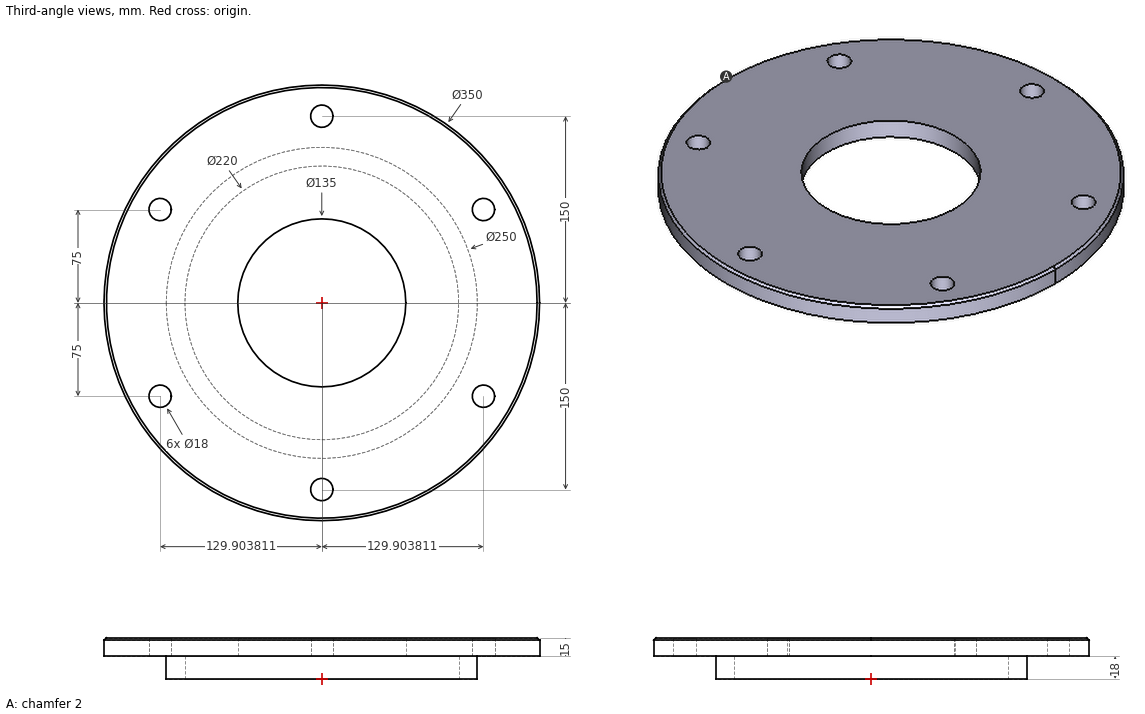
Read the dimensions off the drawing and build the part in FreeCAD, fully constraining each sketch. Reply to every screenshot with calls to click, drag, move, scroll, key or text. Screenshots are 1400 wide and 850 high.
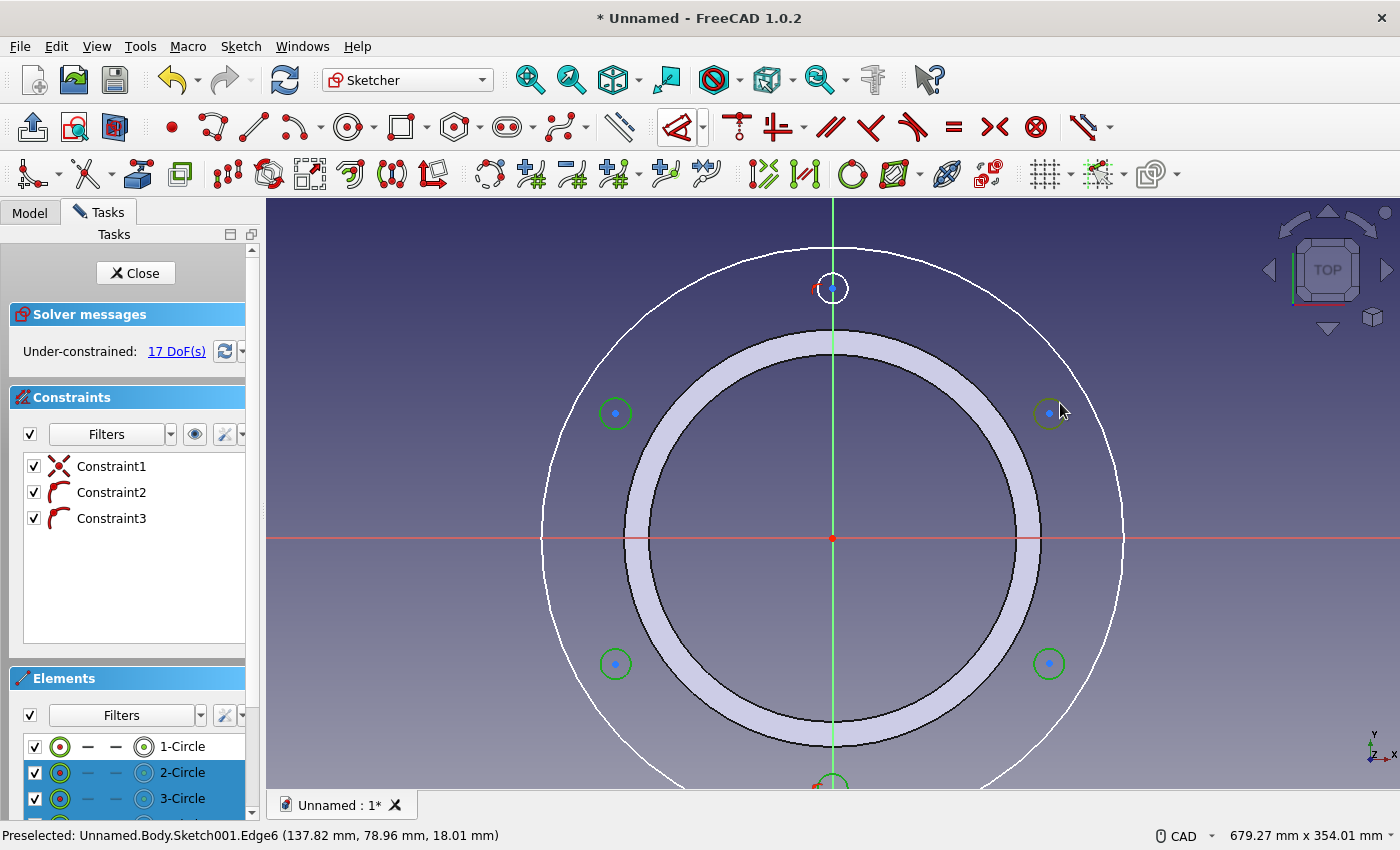
scroll(843, 278, up, 2)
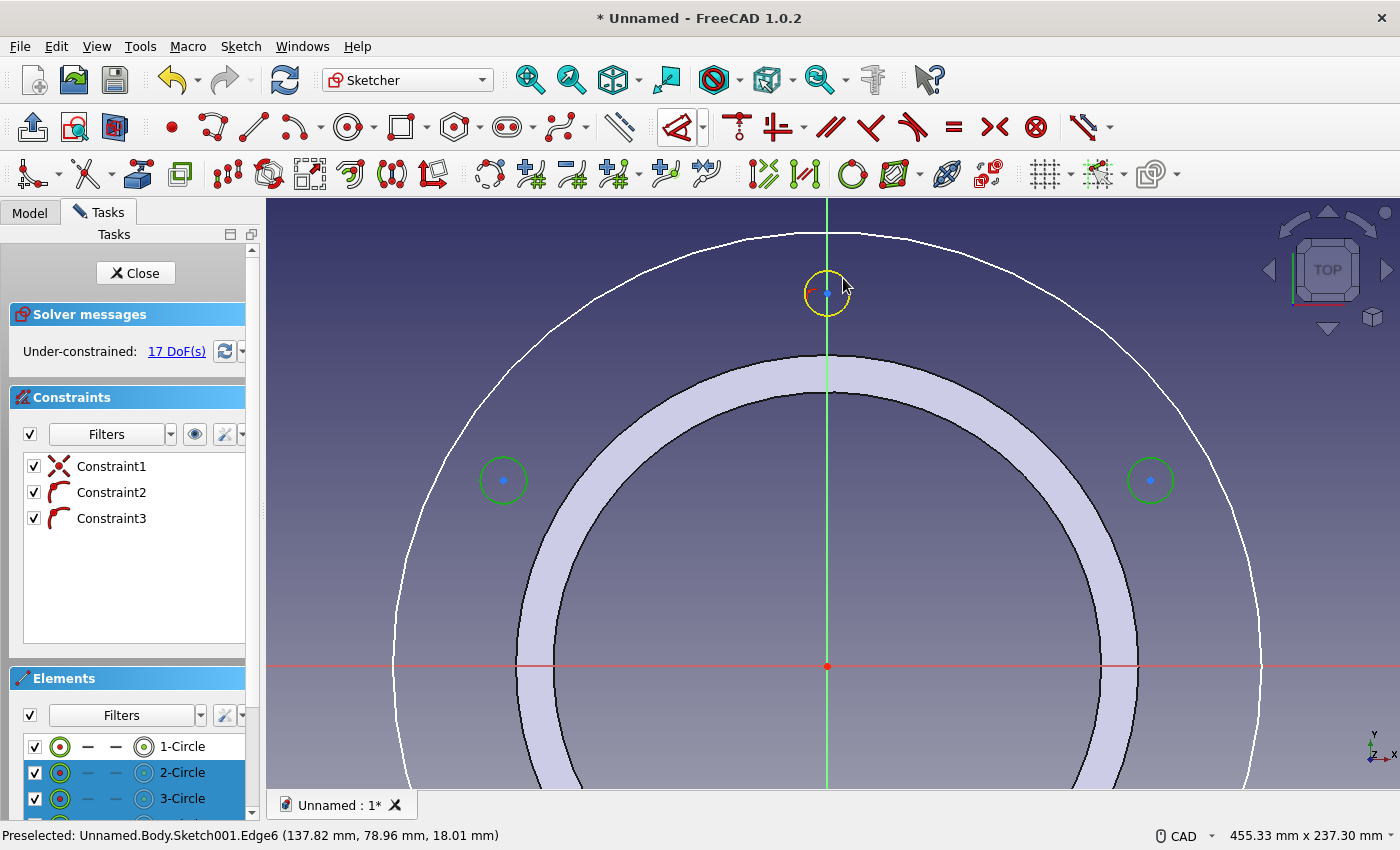
click(843, 277)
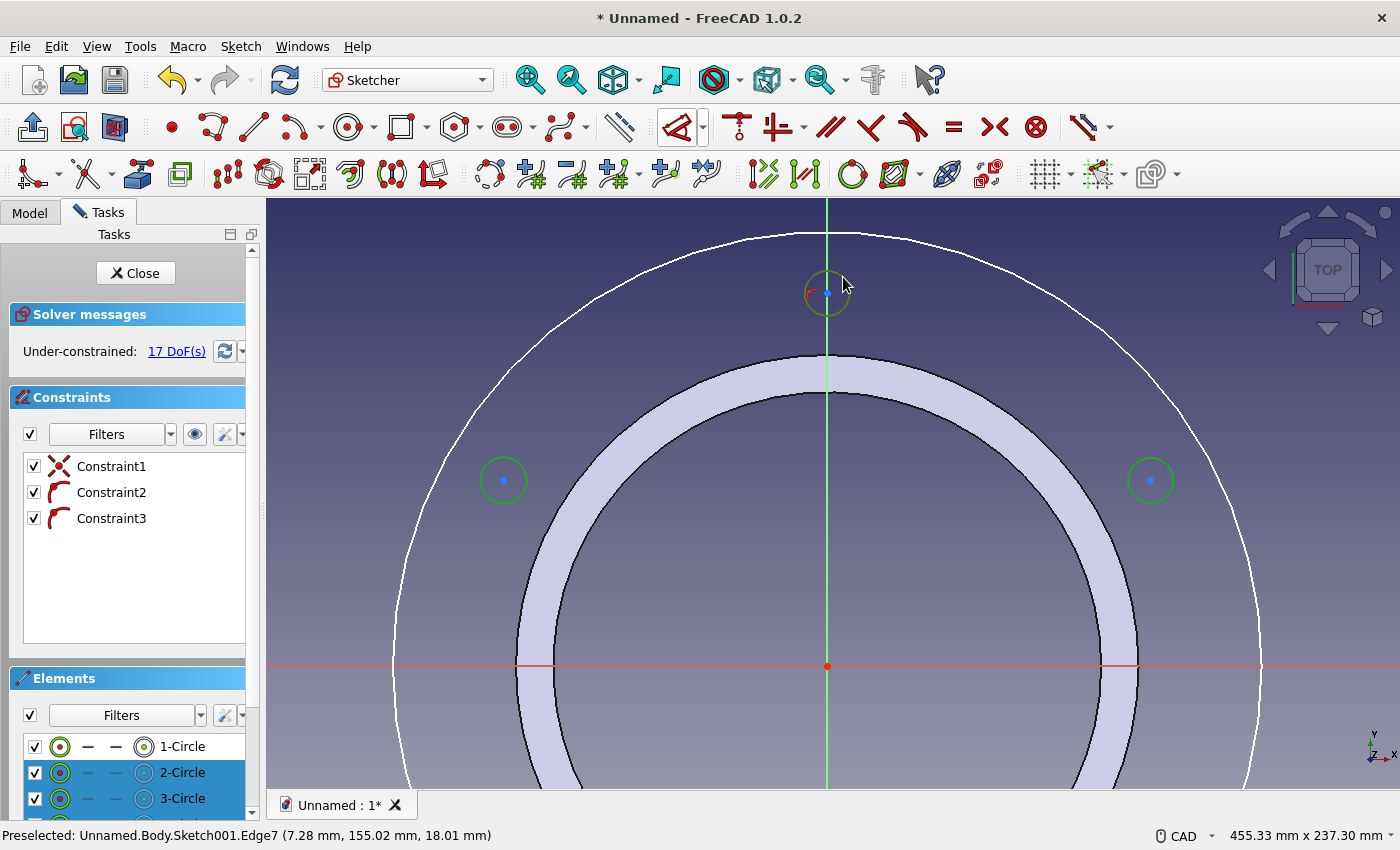
key(e)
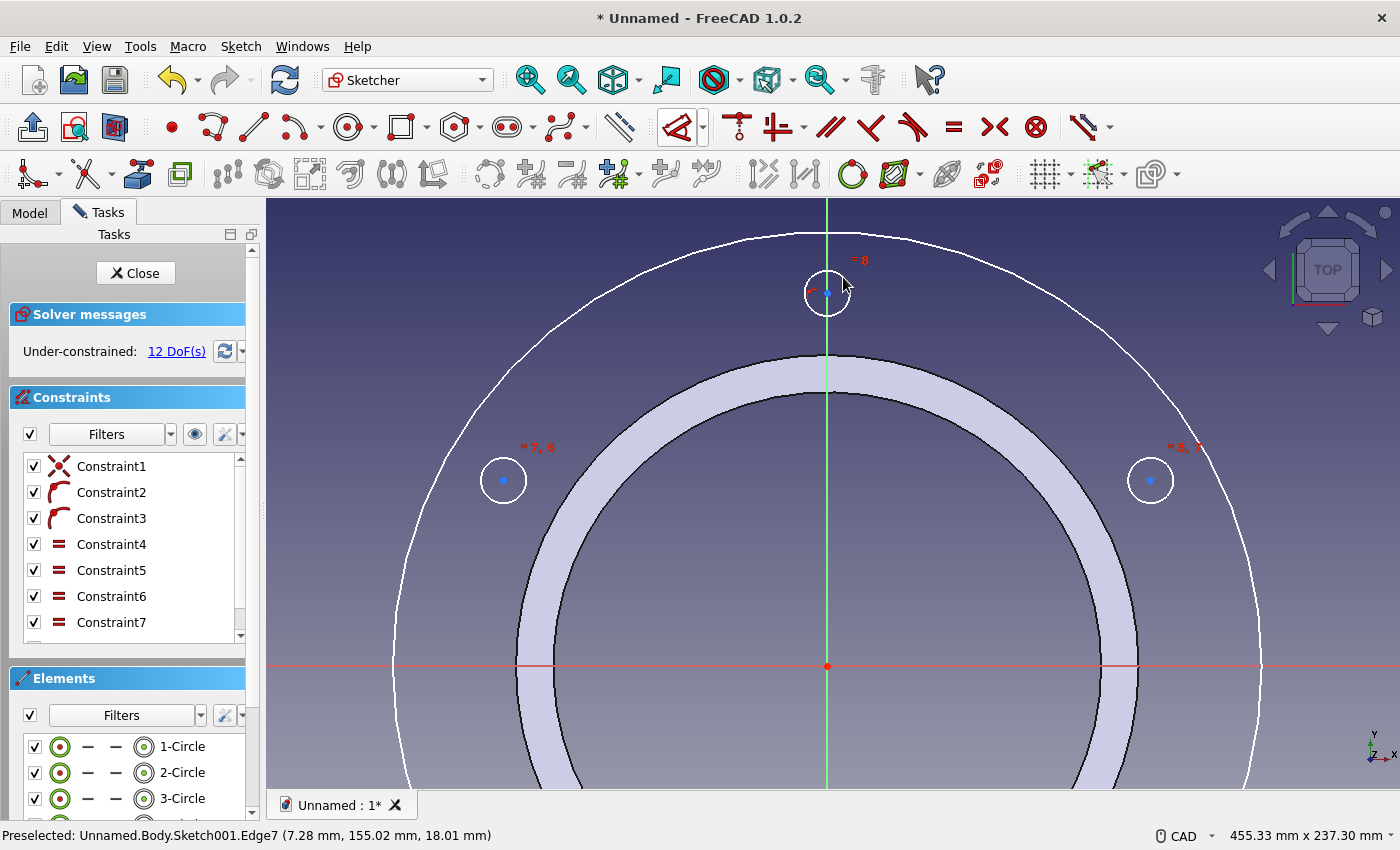
scroll(713, 353, down, 4)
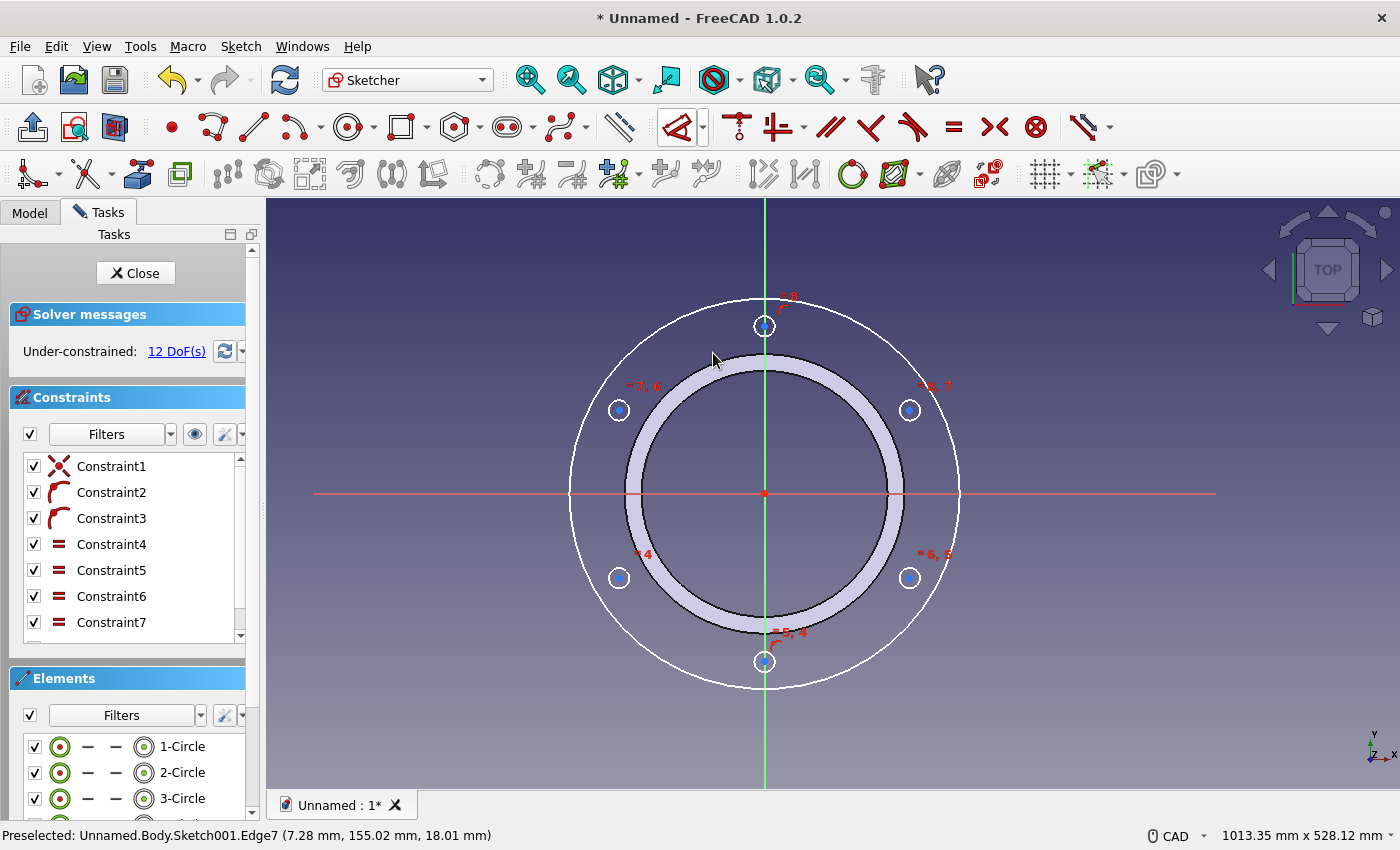
click(619, 578)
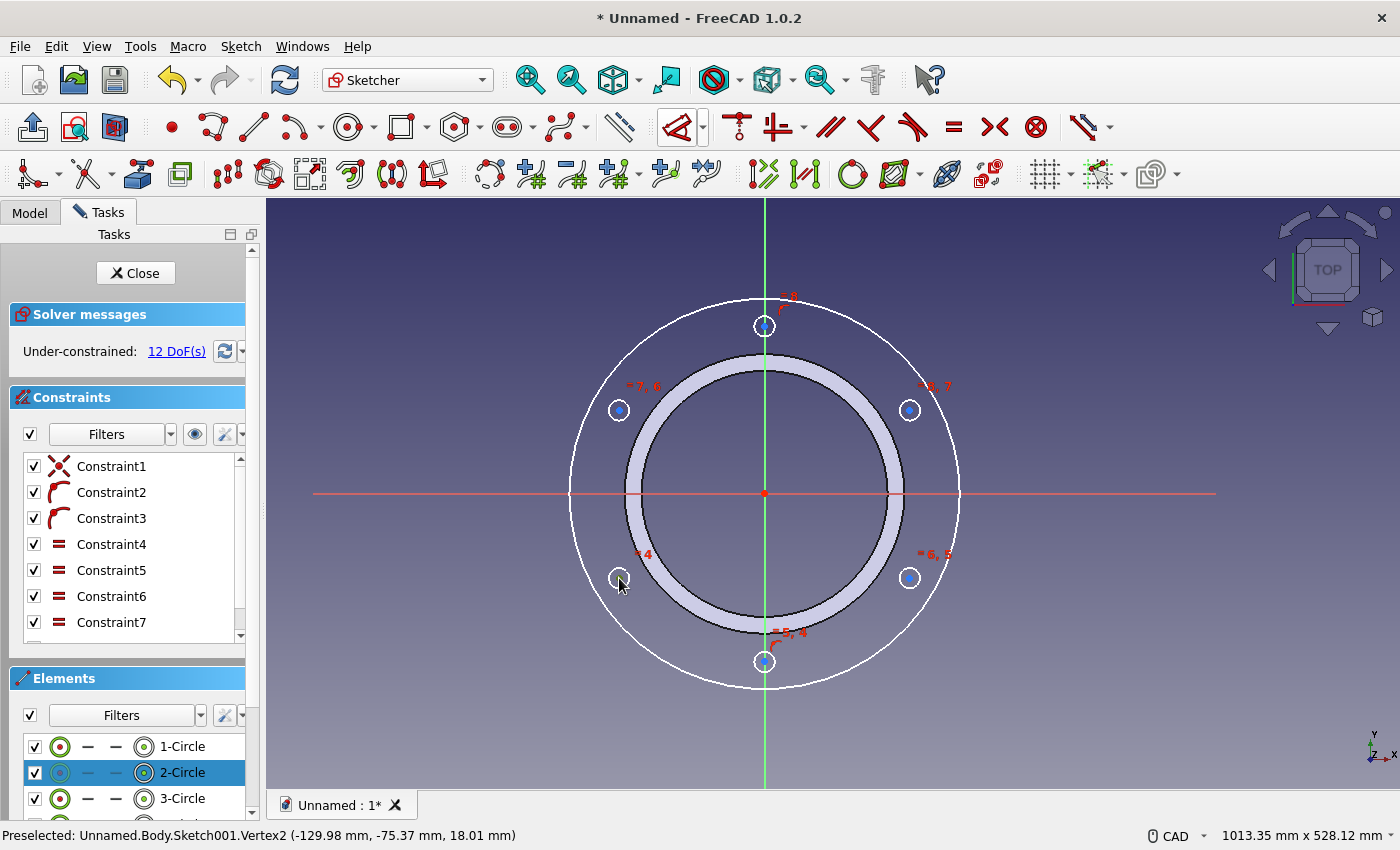
click(910, 578)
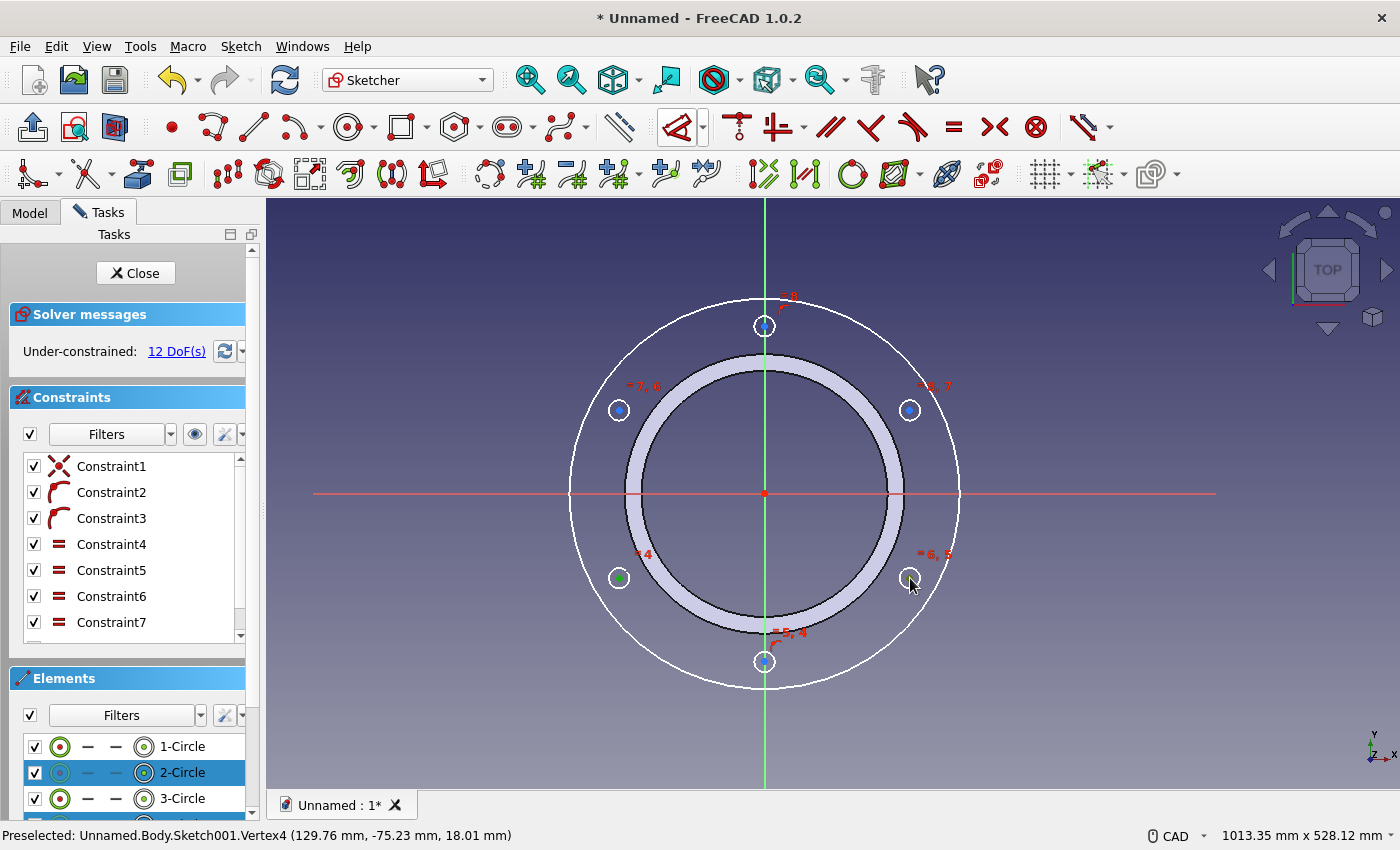
key(h)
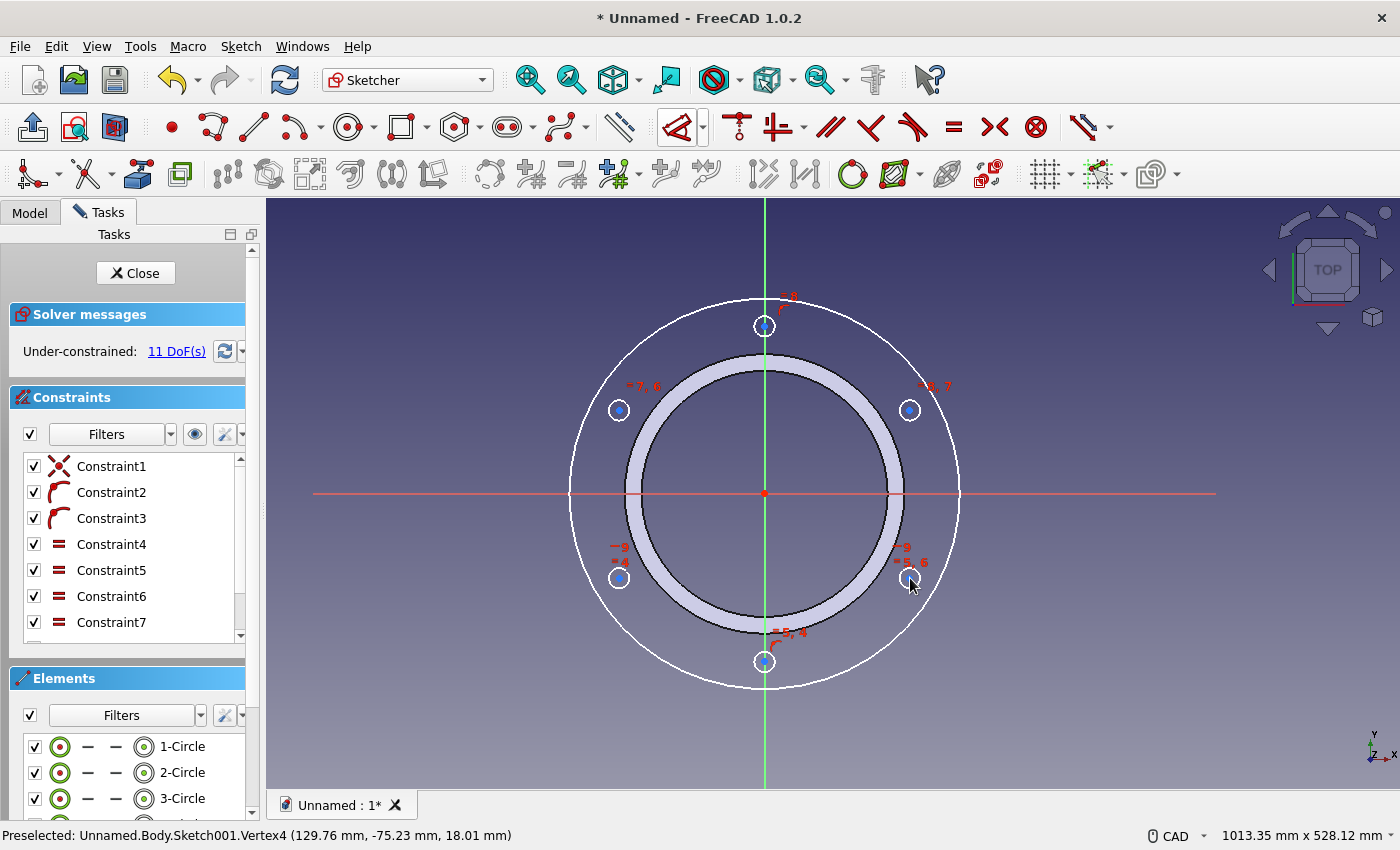
click(619, 578)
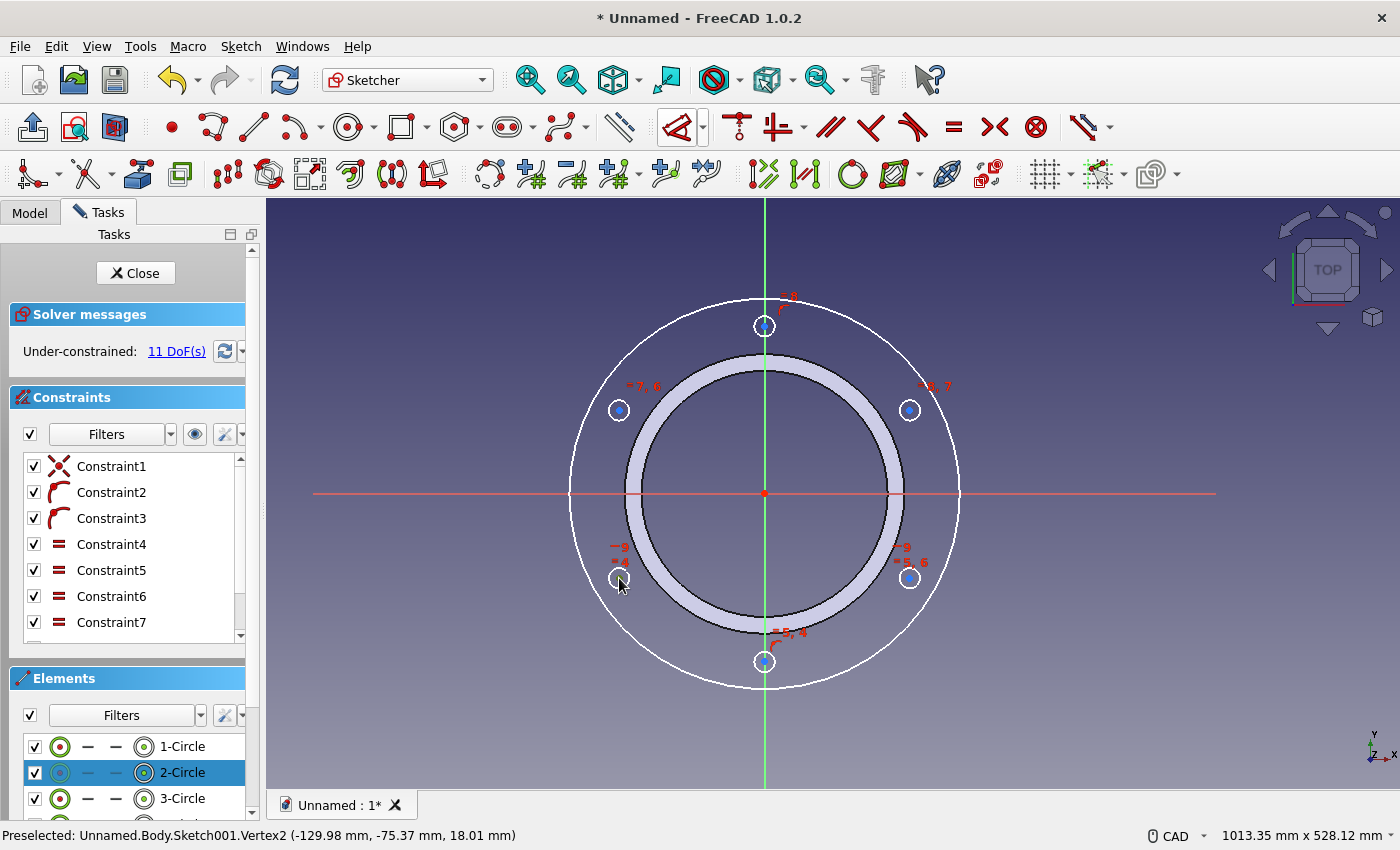
click(619, 410)